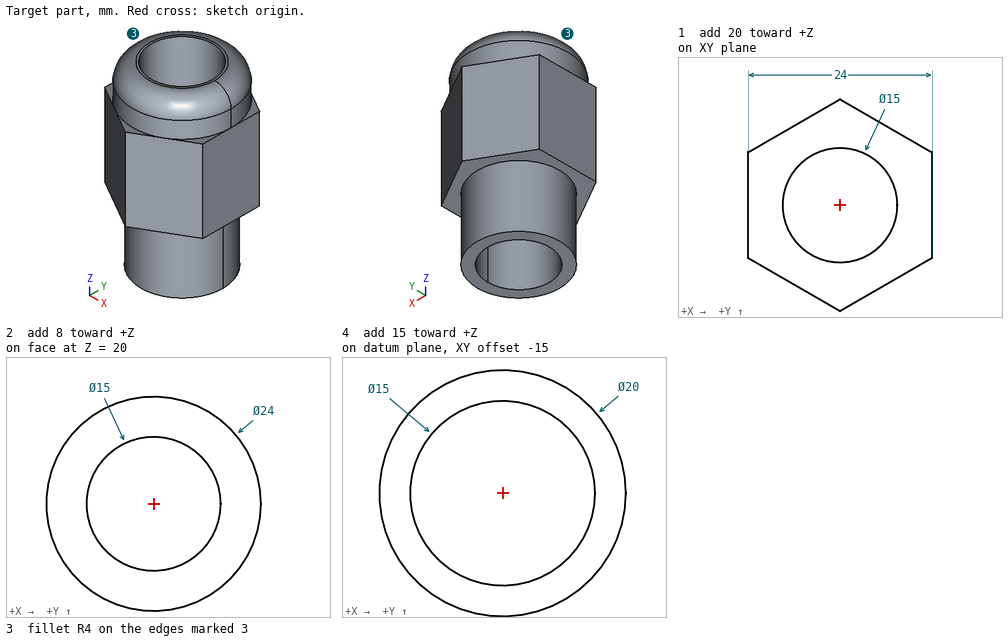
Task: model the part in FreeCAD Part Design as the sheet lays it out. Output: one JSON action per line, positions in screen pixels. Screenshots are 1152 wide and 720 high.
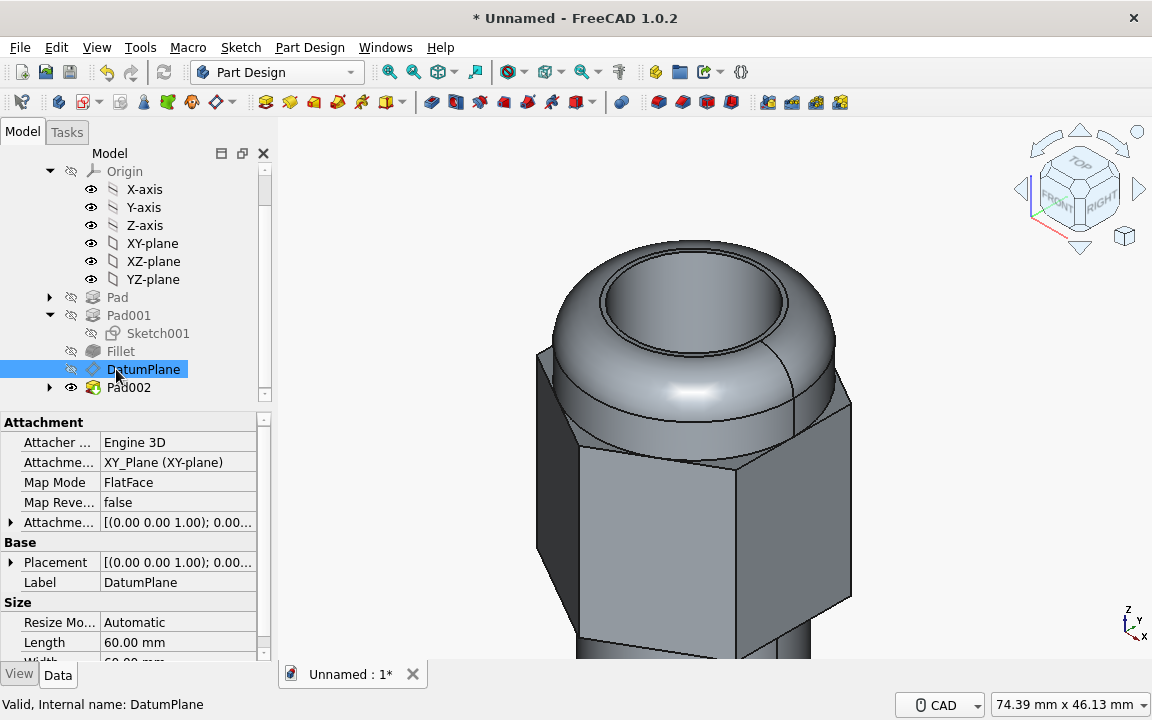
{"action": "key", "text": "v f"}